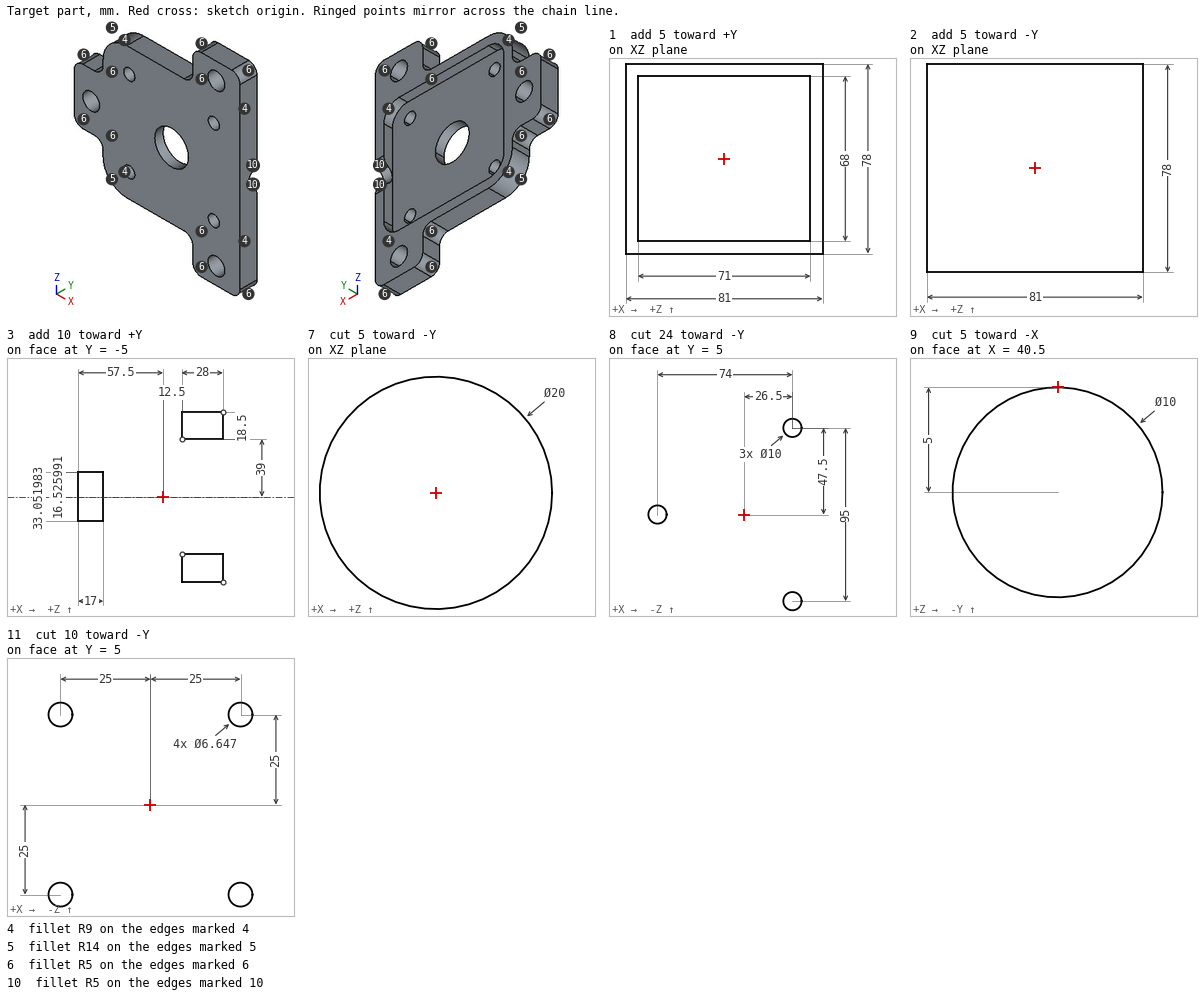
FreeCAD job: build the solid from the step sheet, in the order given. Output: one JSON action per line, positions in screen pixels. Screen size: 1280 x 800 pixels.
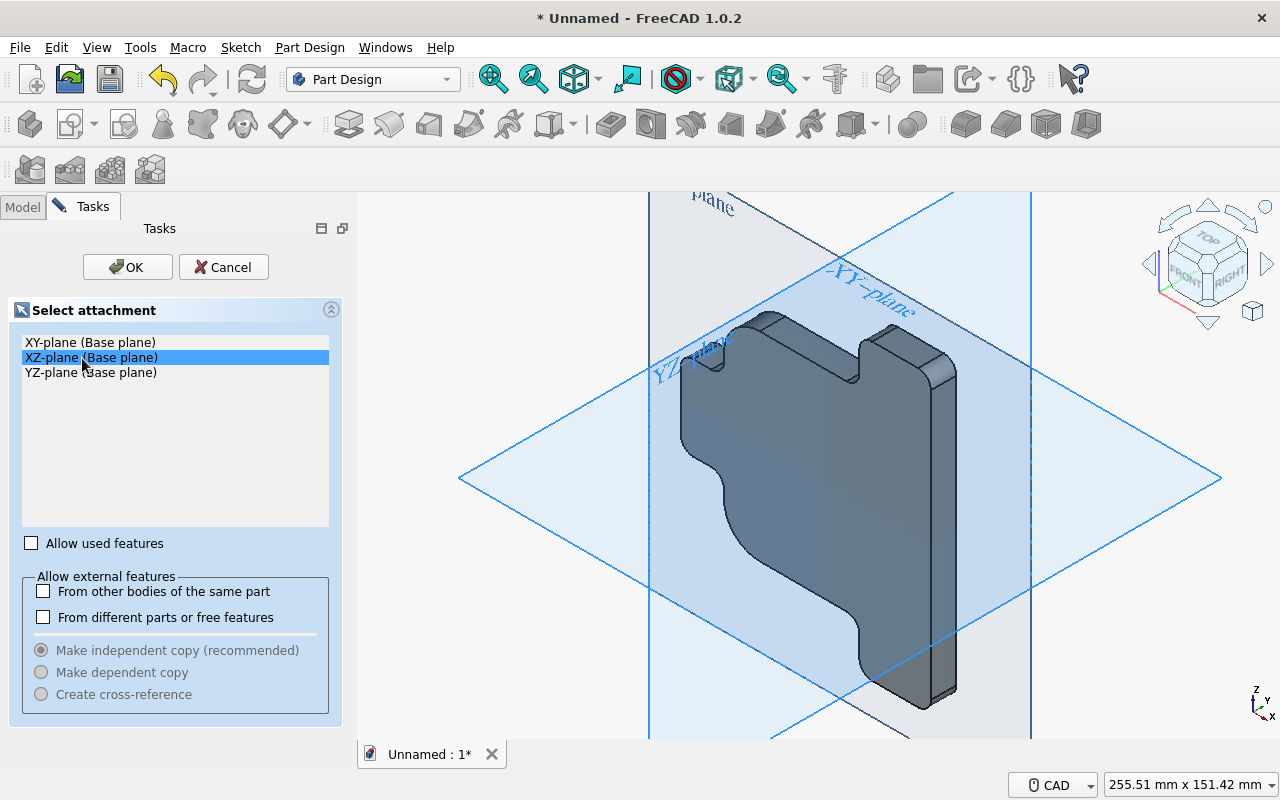
{"action": "left_click", "coordinate": [128, 267]}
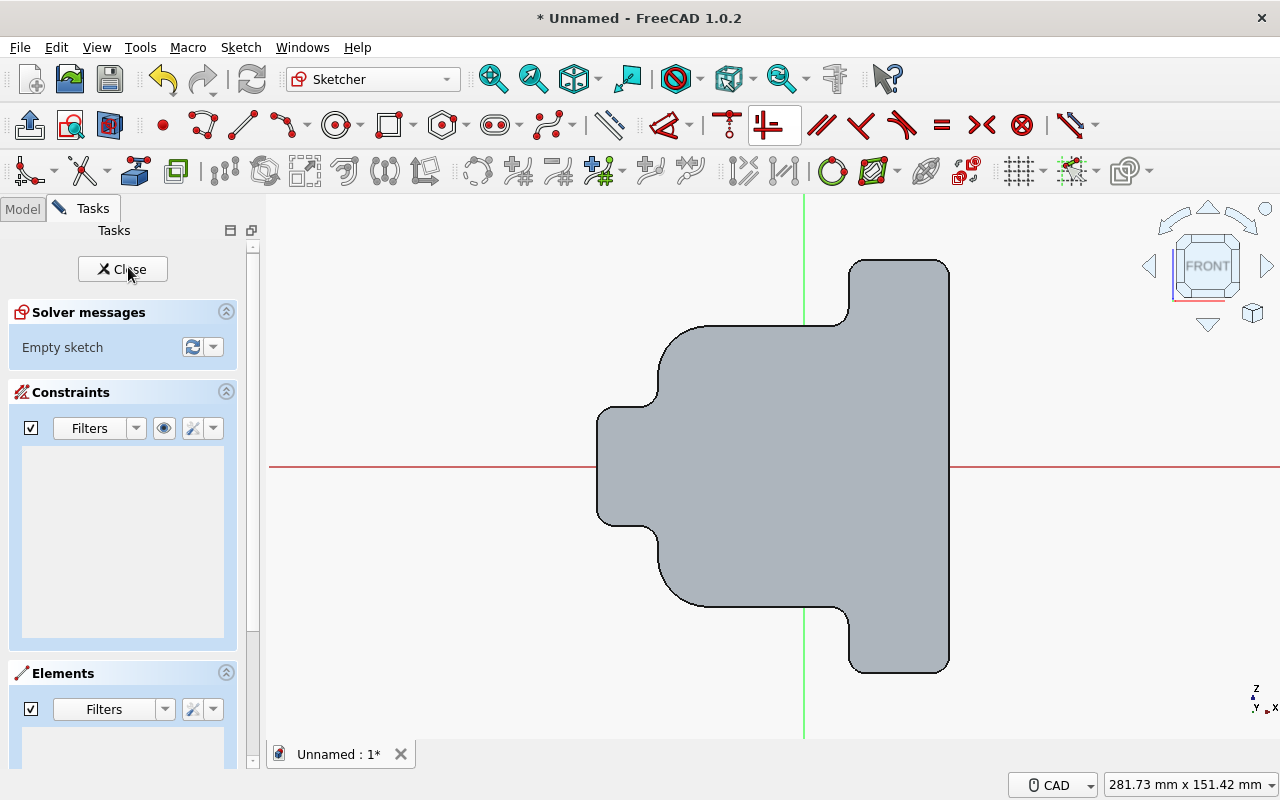
{"action": "key", "text": "q s"}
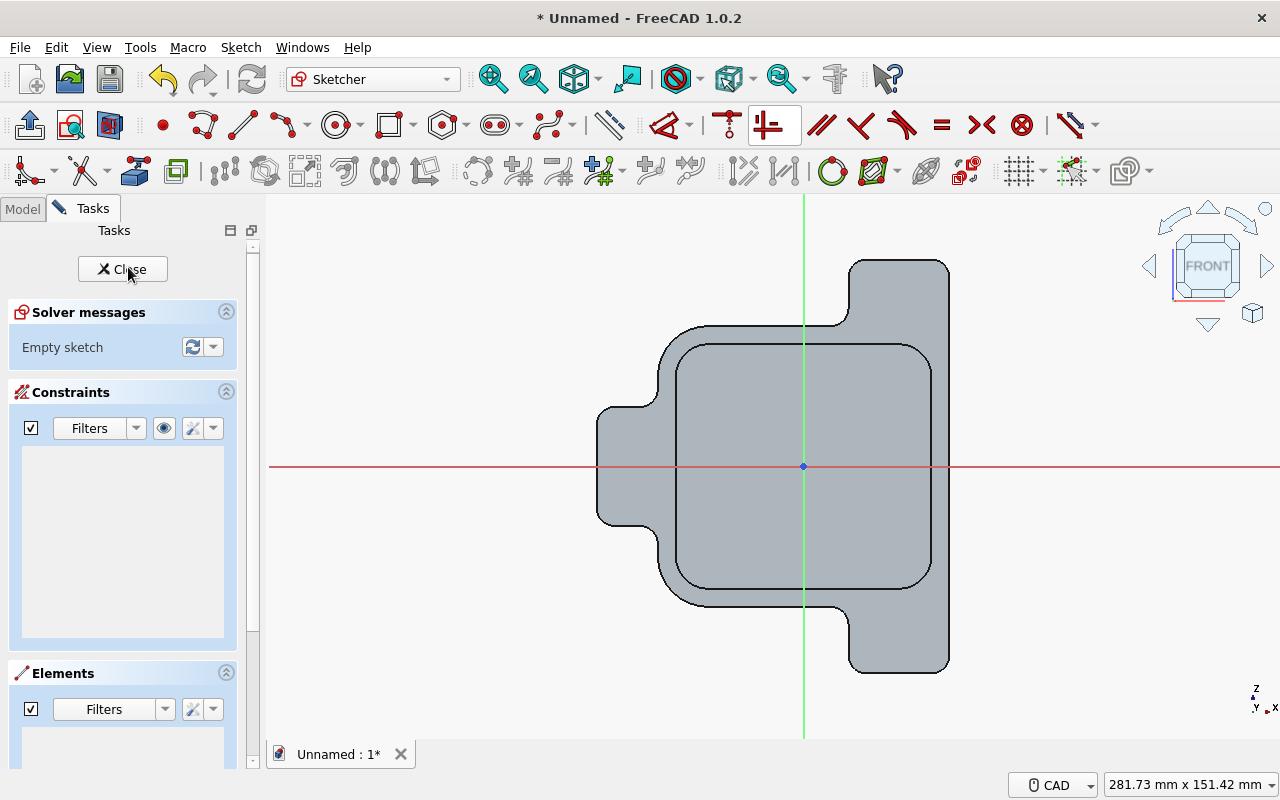
{"action": "scroll", "coordinate": [829, 466], "scroll_direction": "up", "scroll_amount": 8}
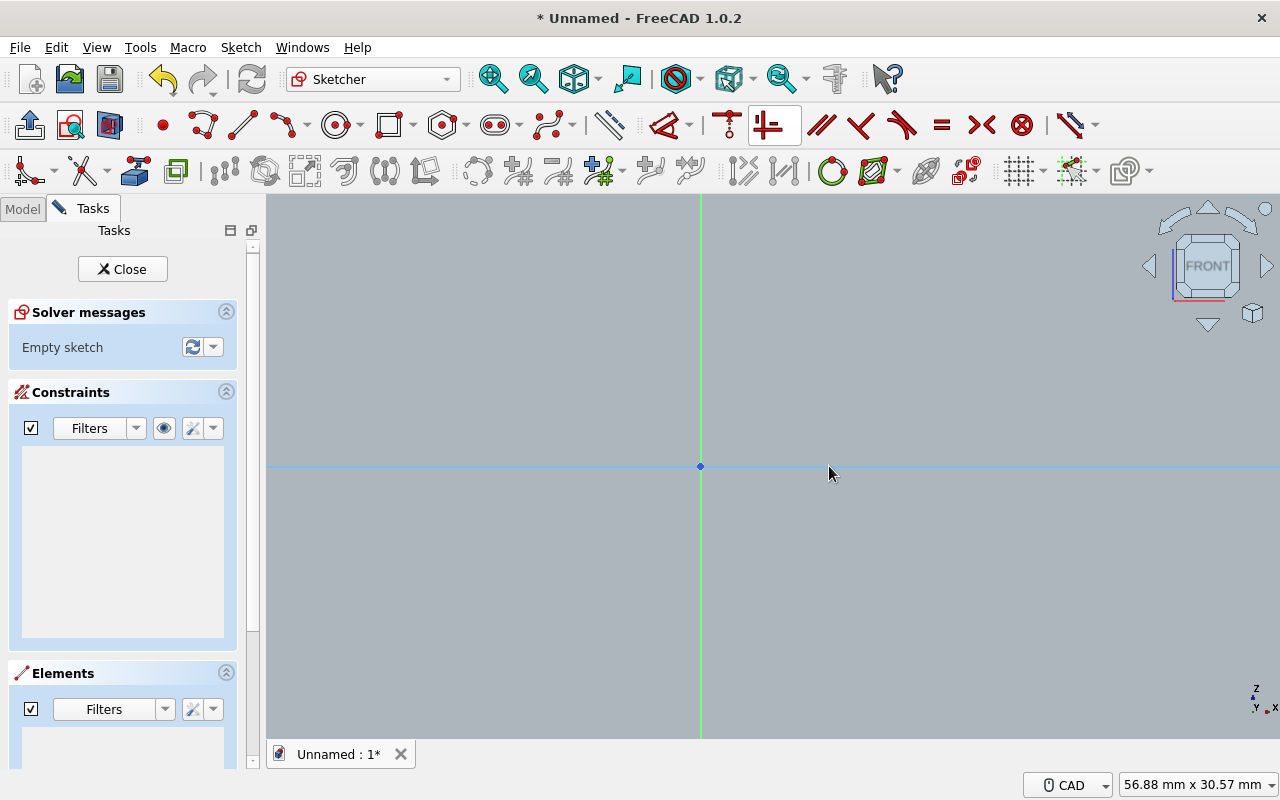
{"action": "key", "text": "g c"}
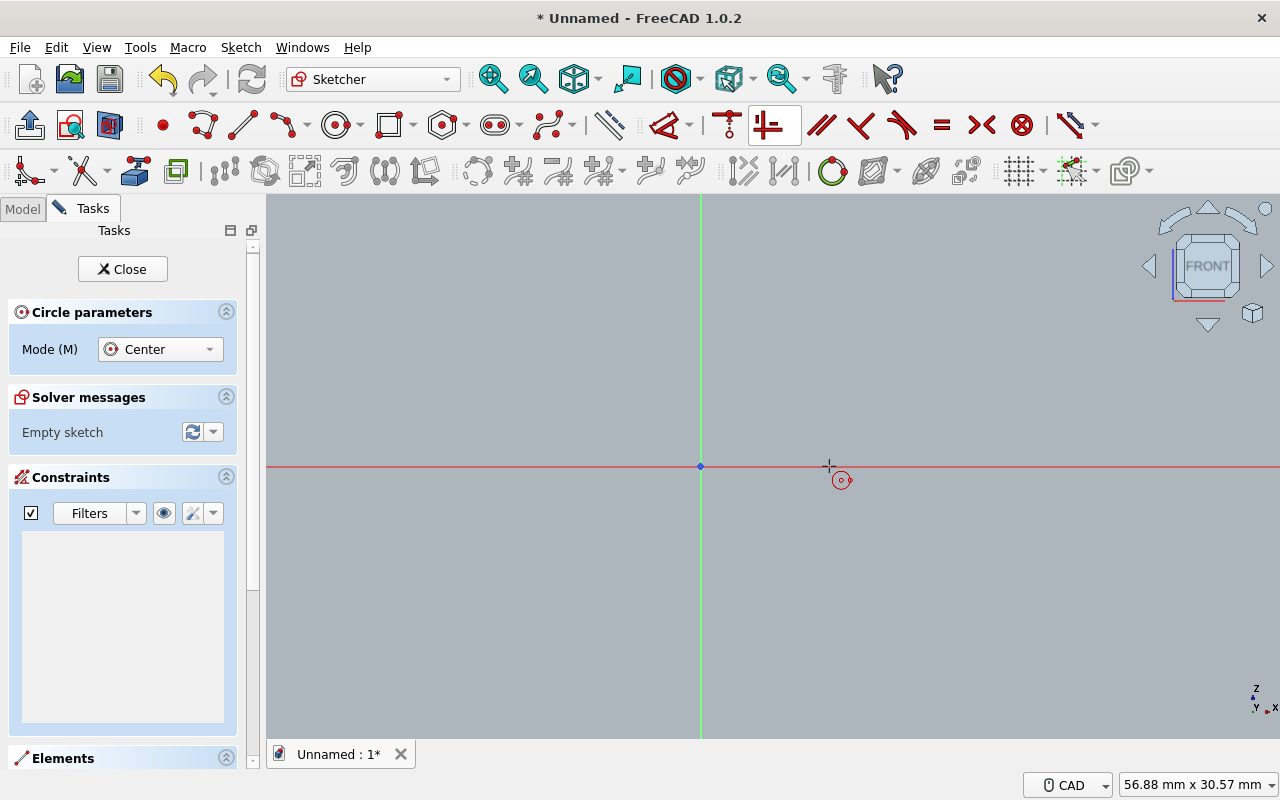
{"action": "left_click", "coordinate": [701, 466]}
{"action": "left_click", "coordinate": [827, 340]}
{"action": "key", "text": "Escape"}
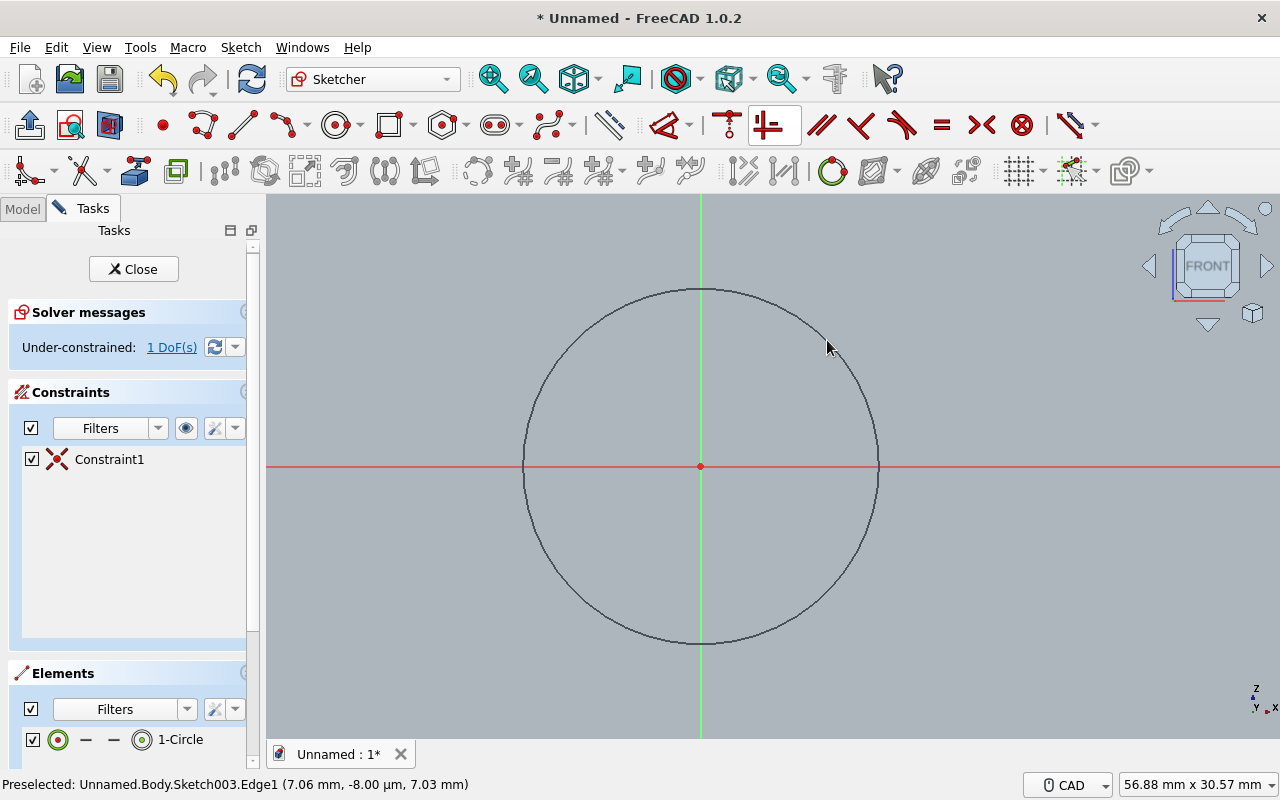
{"action": "key", "text": "d"}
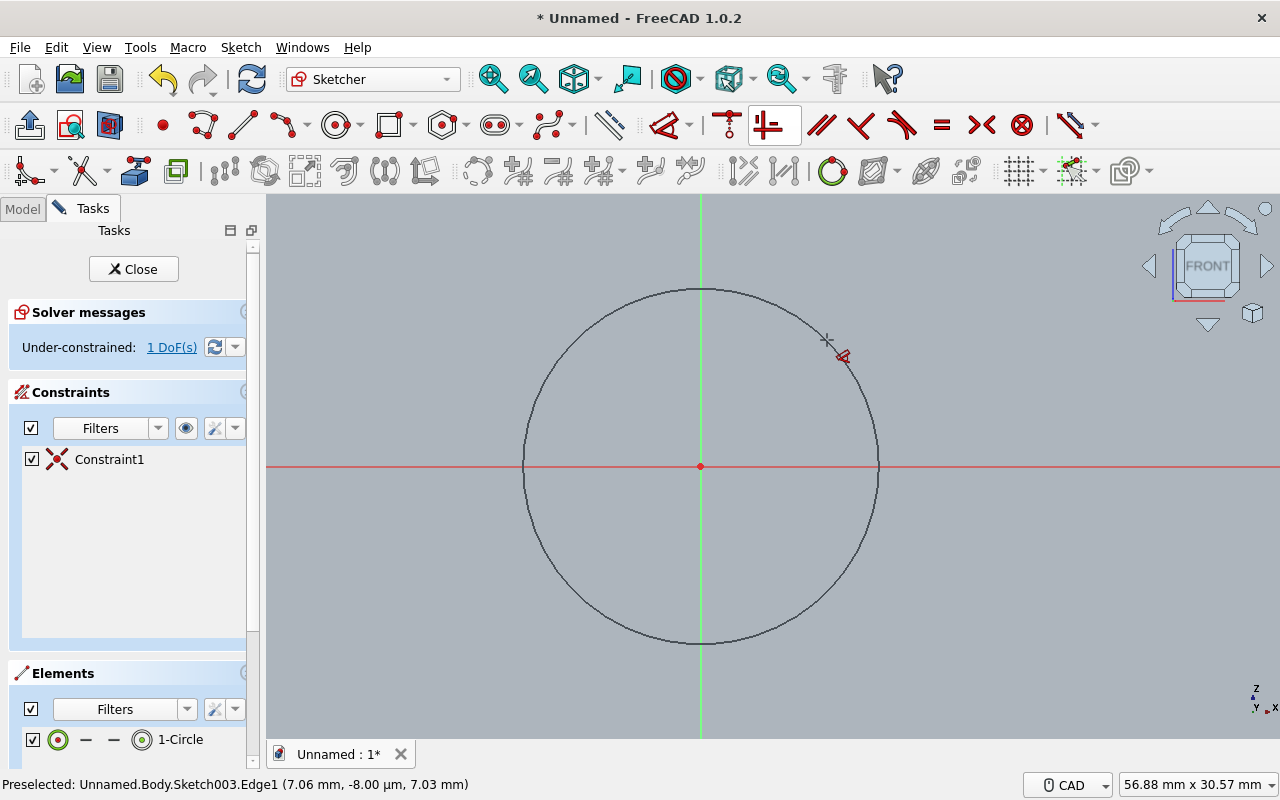
{"action": "left_click", "coordinate": [826, 340]}
{"action": "left_click", "coordinate": [848, 317]}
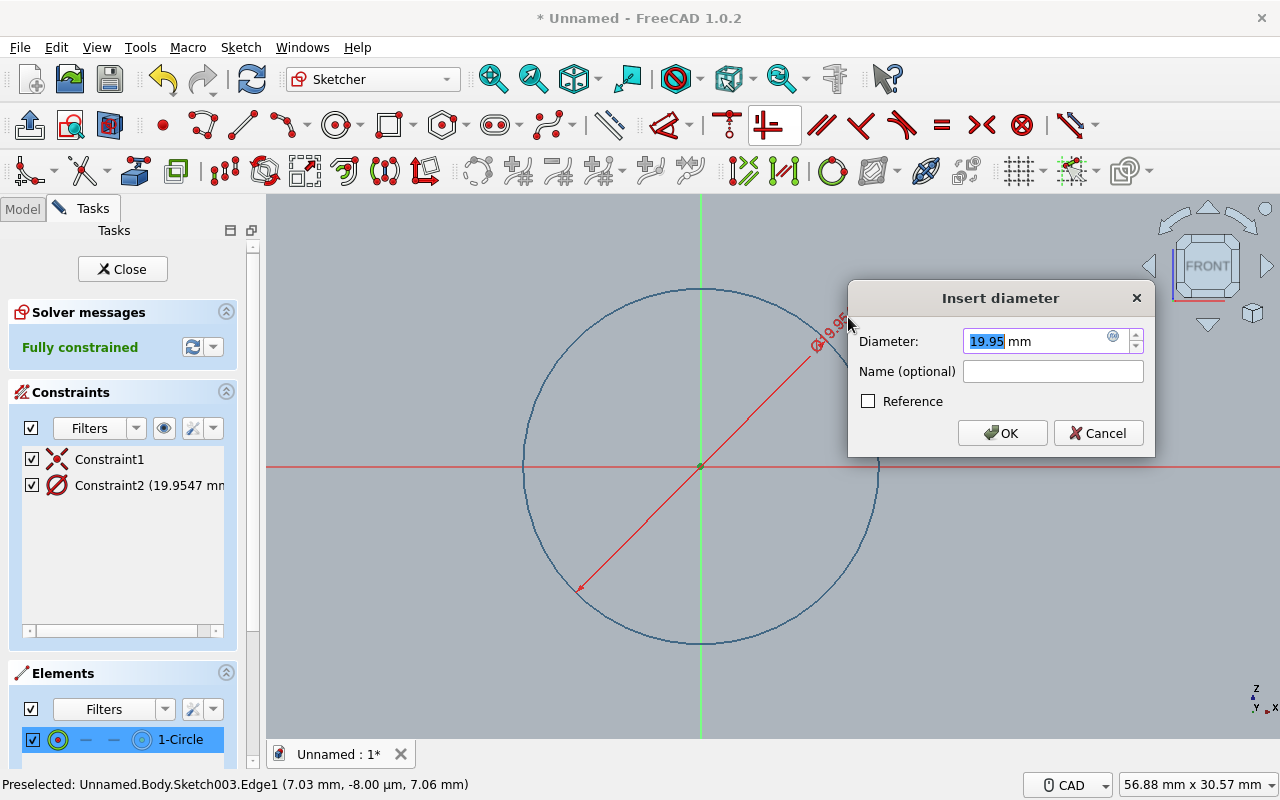
{"action": "type", "text": "20"}
{"action": "key", "text": "Return"}
{"action": "key", "text": "Escape"}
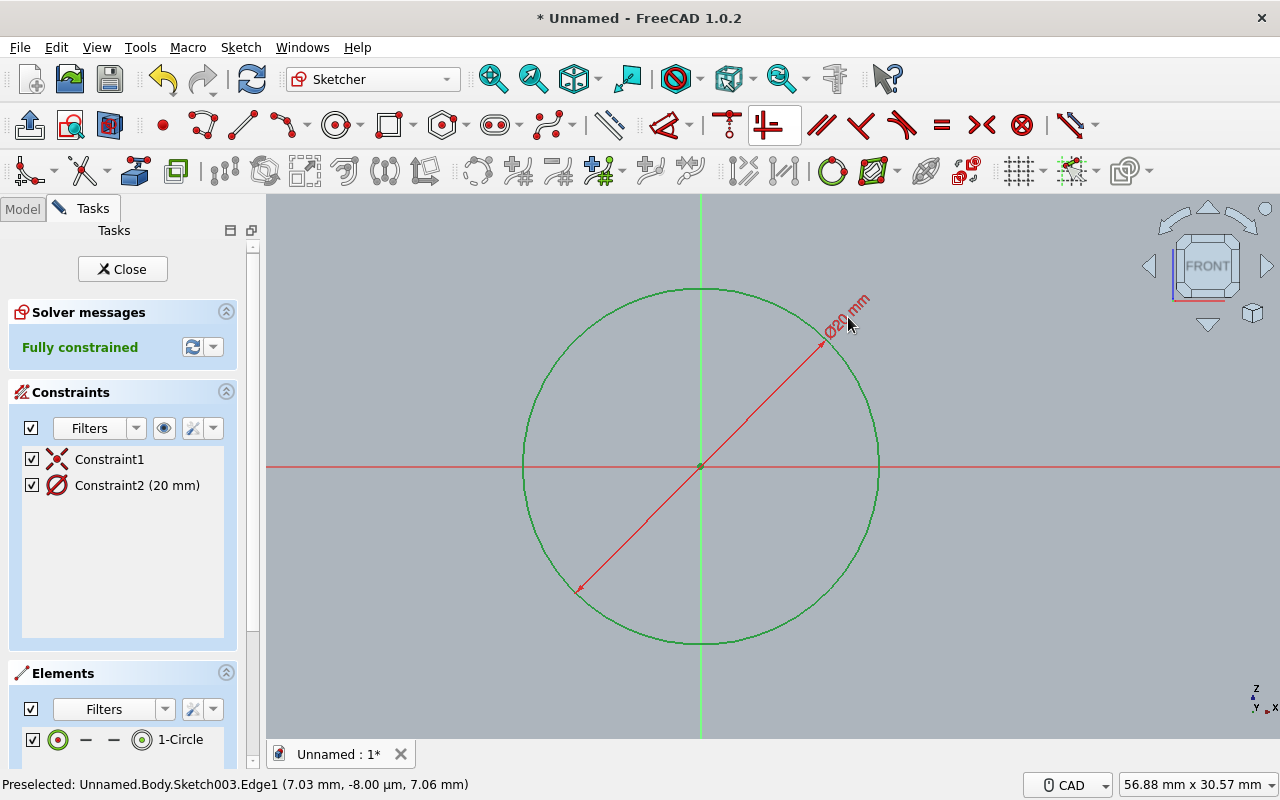
{"action": "left_click", "coordinate": [123, 269]}